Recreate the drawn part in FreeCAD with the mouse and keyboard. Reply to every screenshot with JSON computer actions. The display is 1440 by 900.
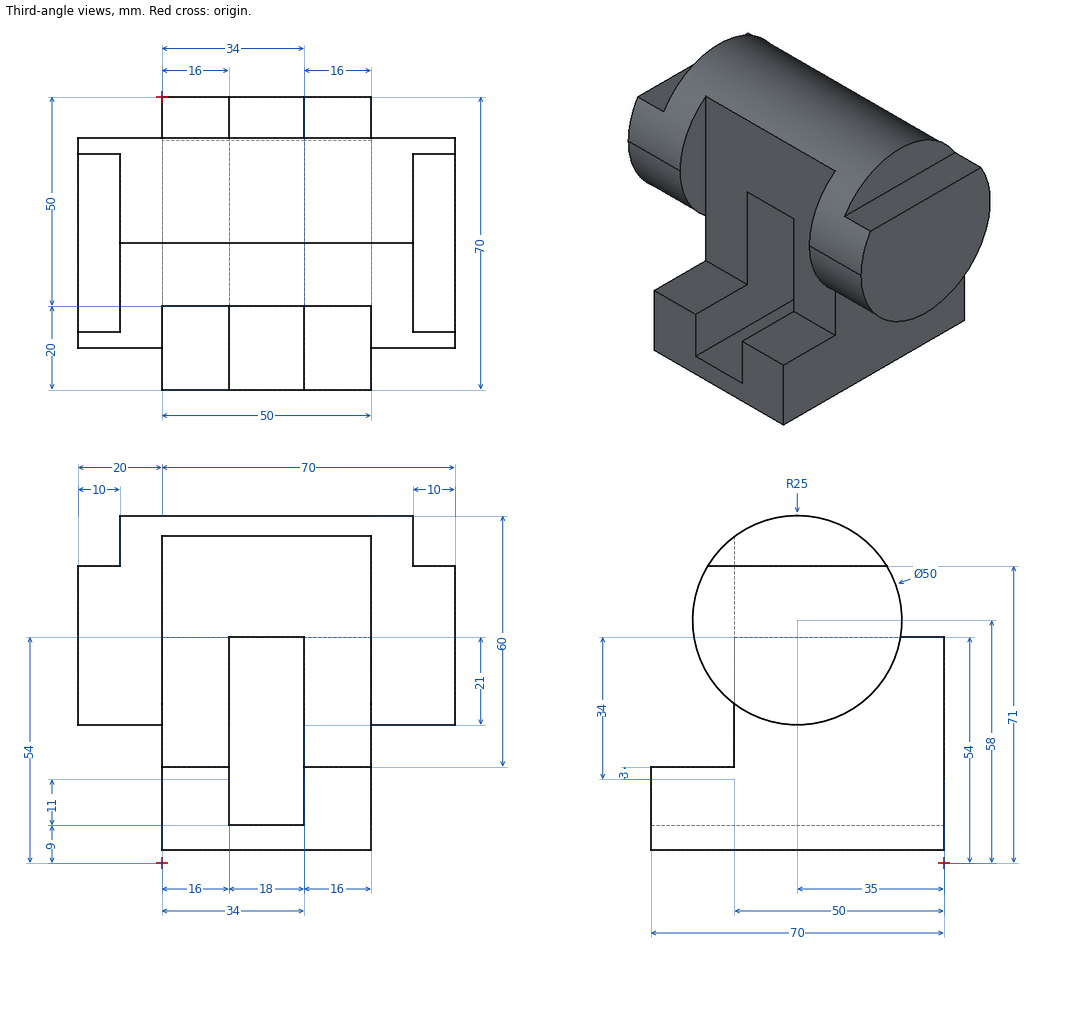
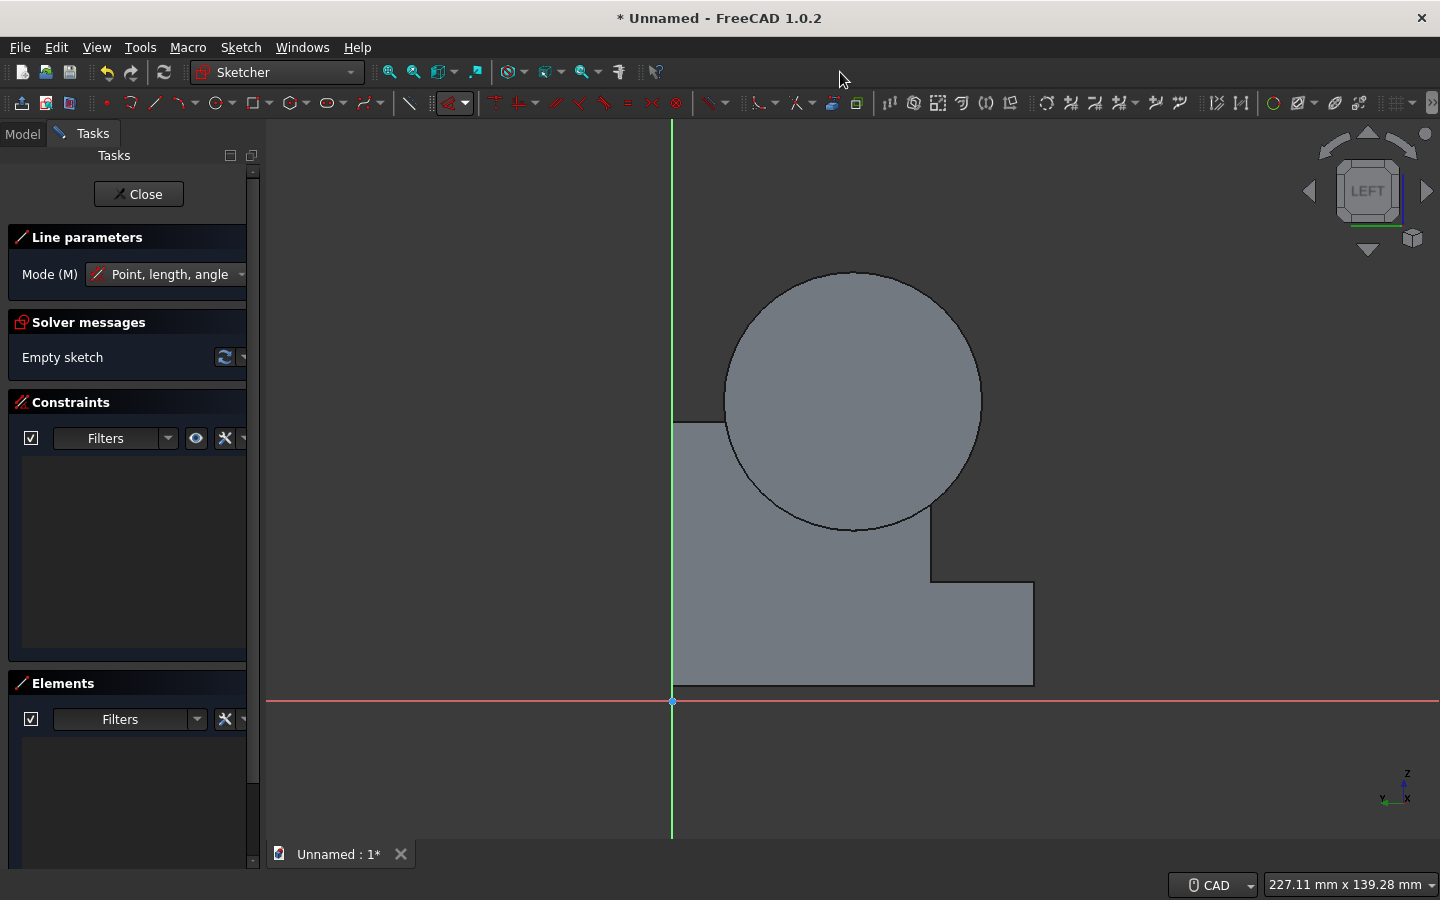
{"action": "left_click", "coordinate": [743, 334]}
{"action": "left_click", "coordinate": [963, 334]}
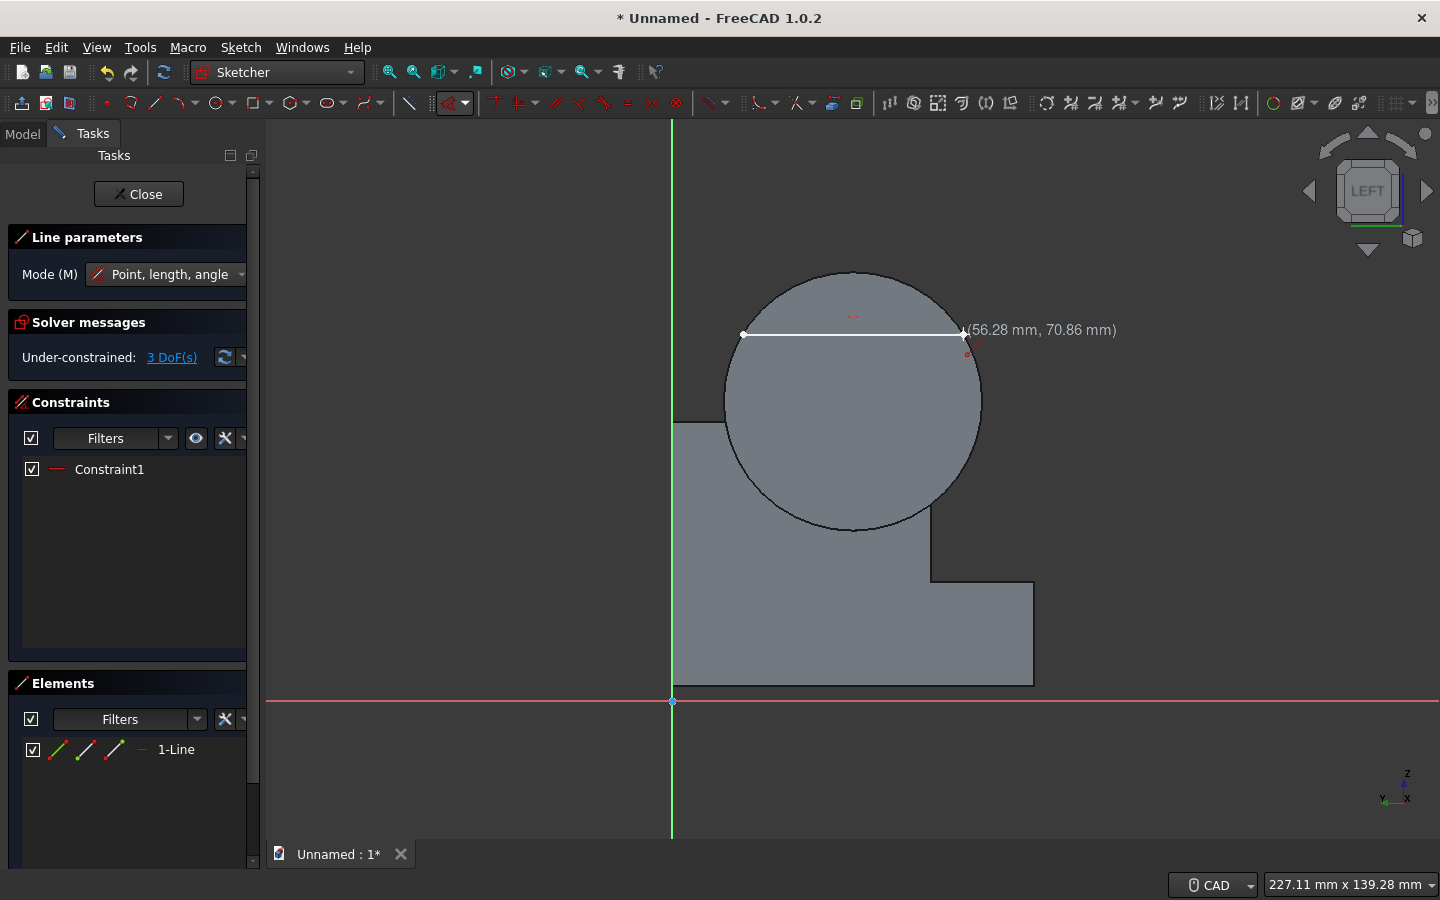
{"action": "key", "text": "g 3 a"}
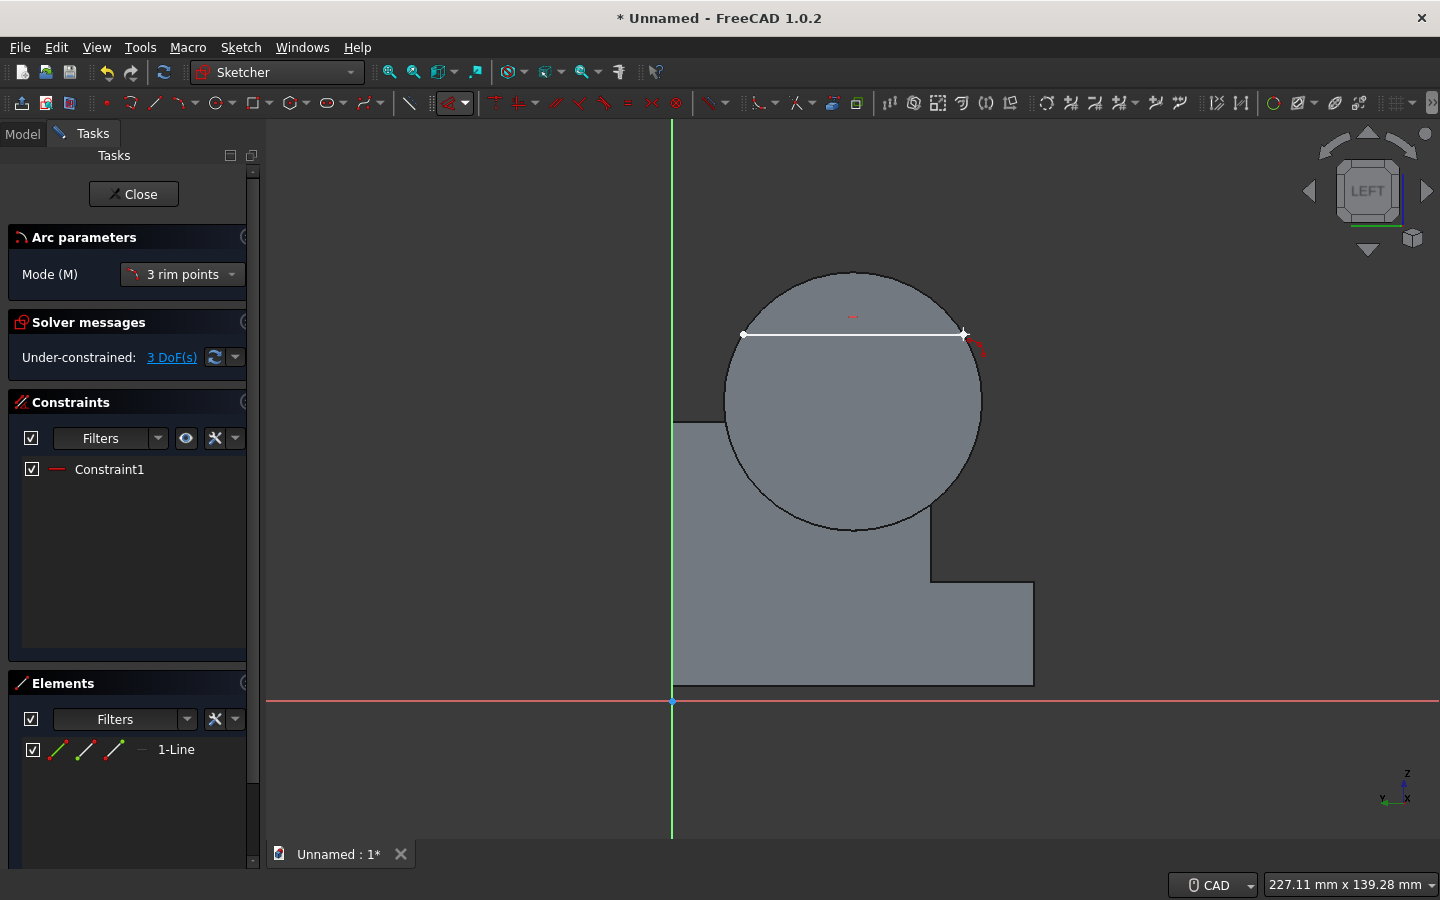
{"action": "left_click", "coordinate": [963, 335]}
{"action": "left_click", "coordinate": [743, 335]}
{"action": "left_click", "coordinate": [853, 272]}
{"action": "key", "text": "Escape"}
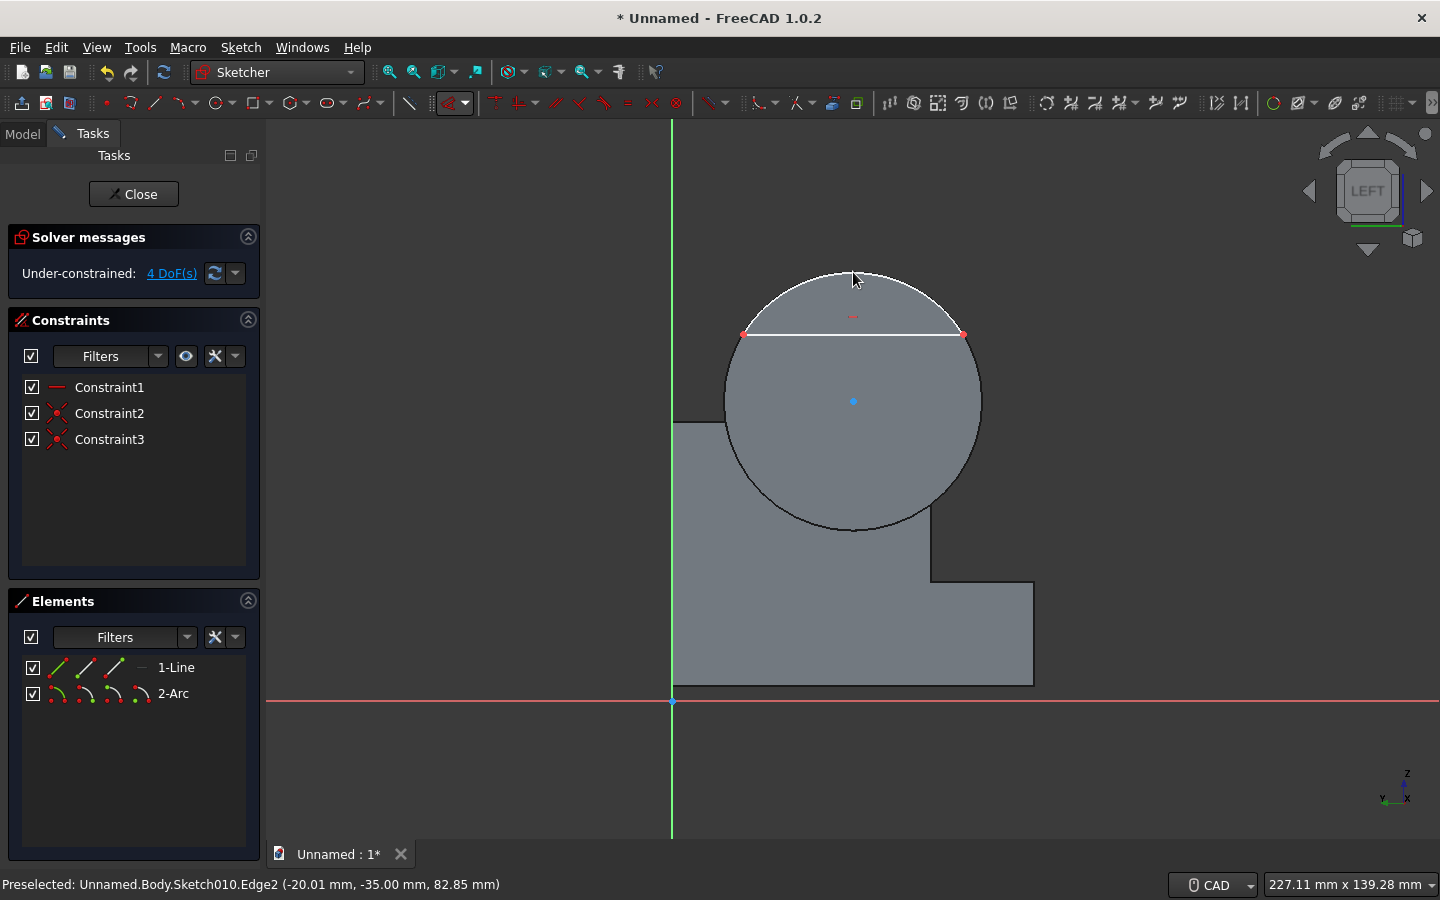
{"action": "left_click", "coordinate": [904, 284]}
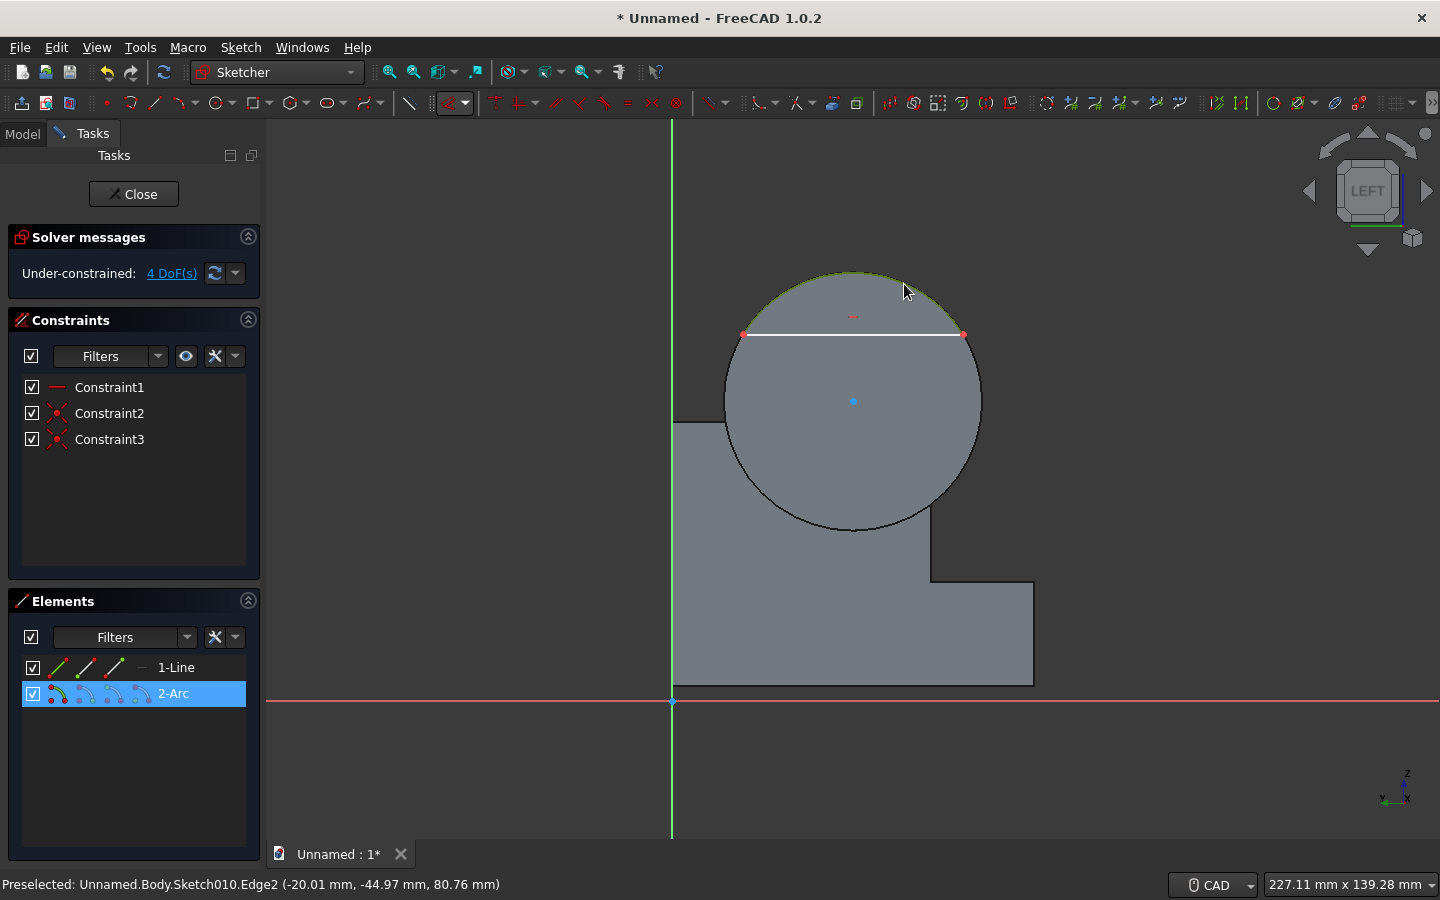
{"action": "key", "text": "k r"}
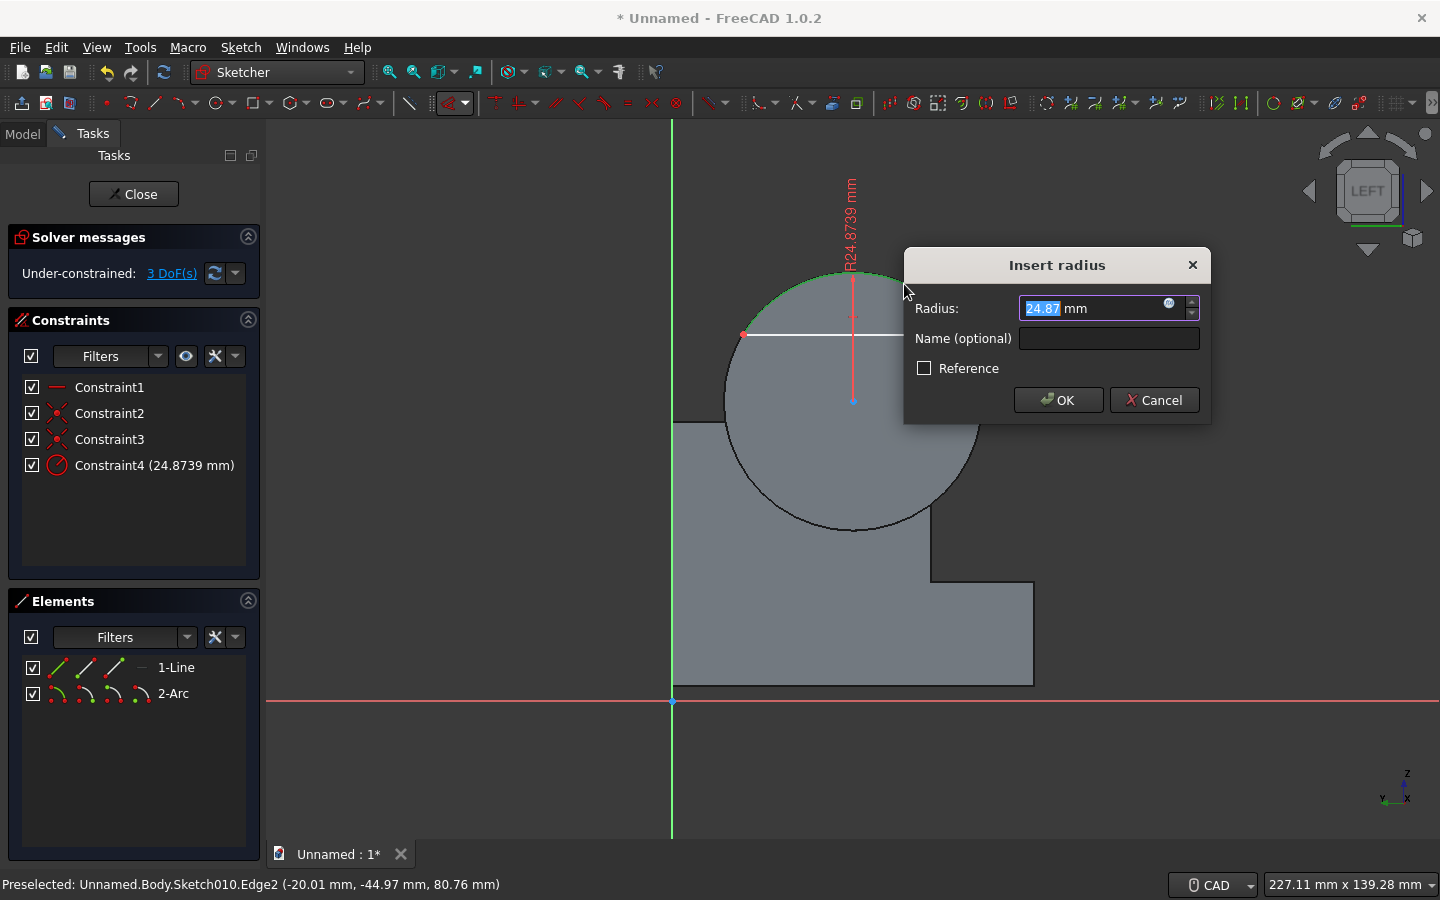
{"action": "type", "text": "25"}
{"action": "key", "text": "Return"}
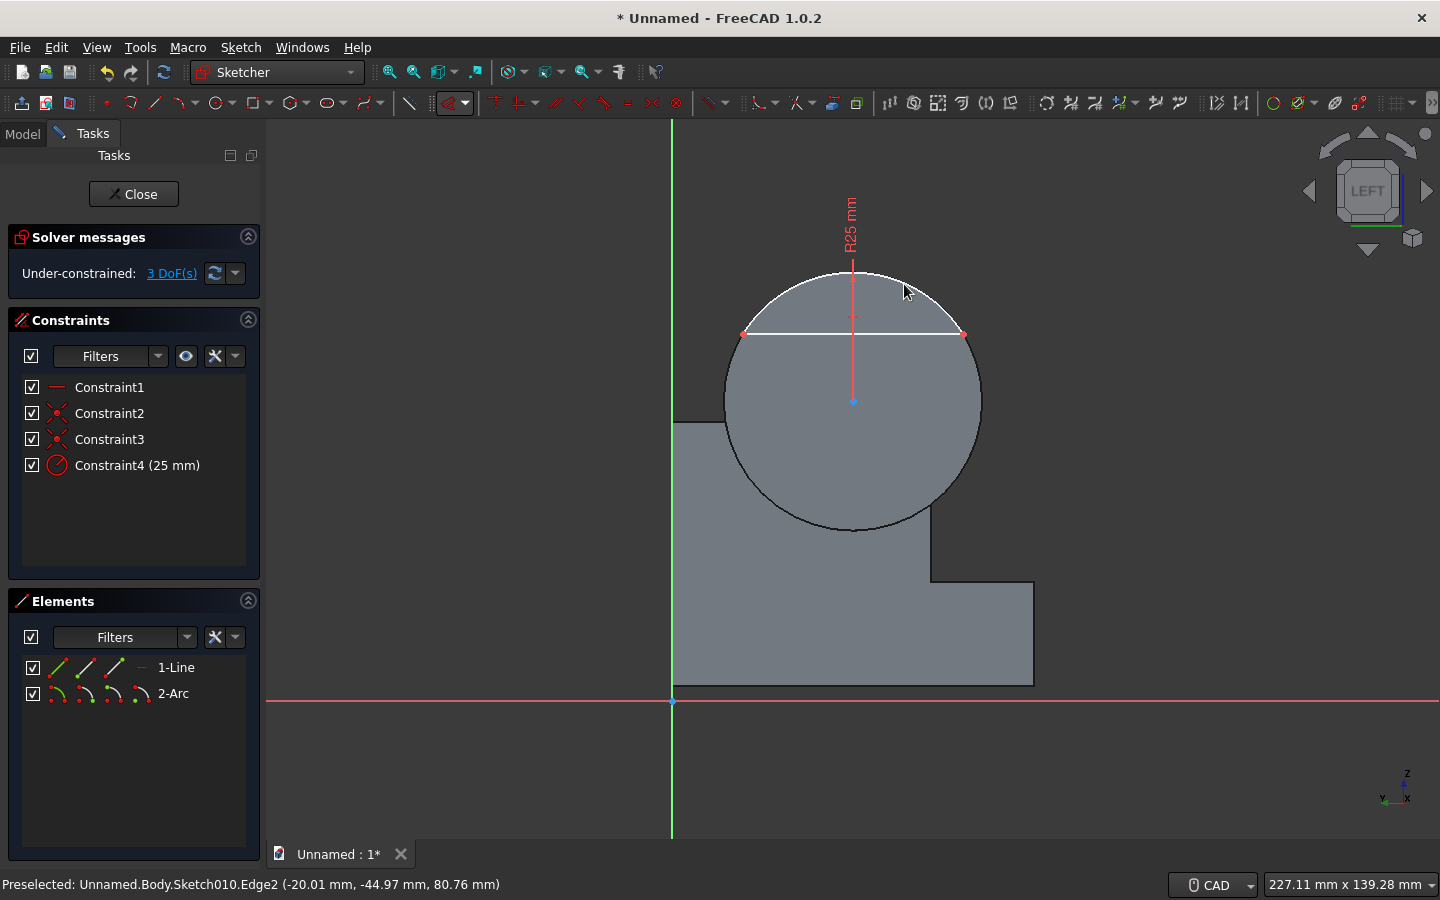
{"action": "left_click", "coordinate": [743, 334]}